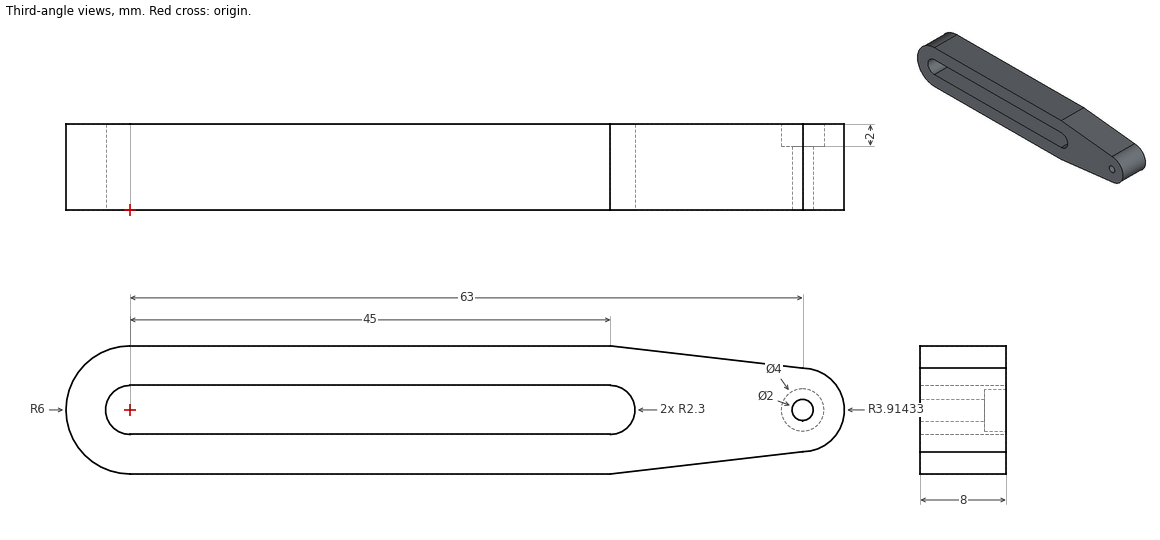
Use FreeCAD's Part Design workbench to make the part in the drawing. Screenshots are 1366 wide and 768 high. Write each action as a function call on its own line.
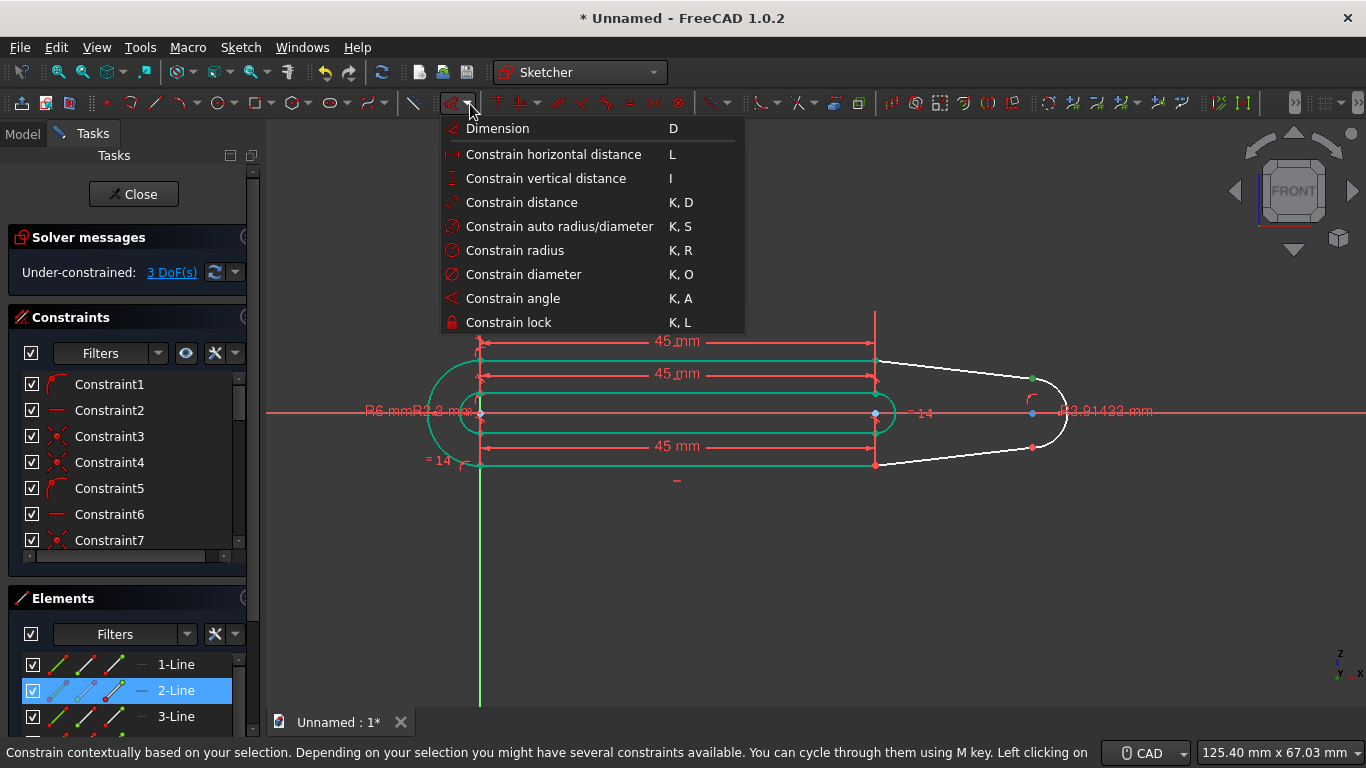
click(593, 154)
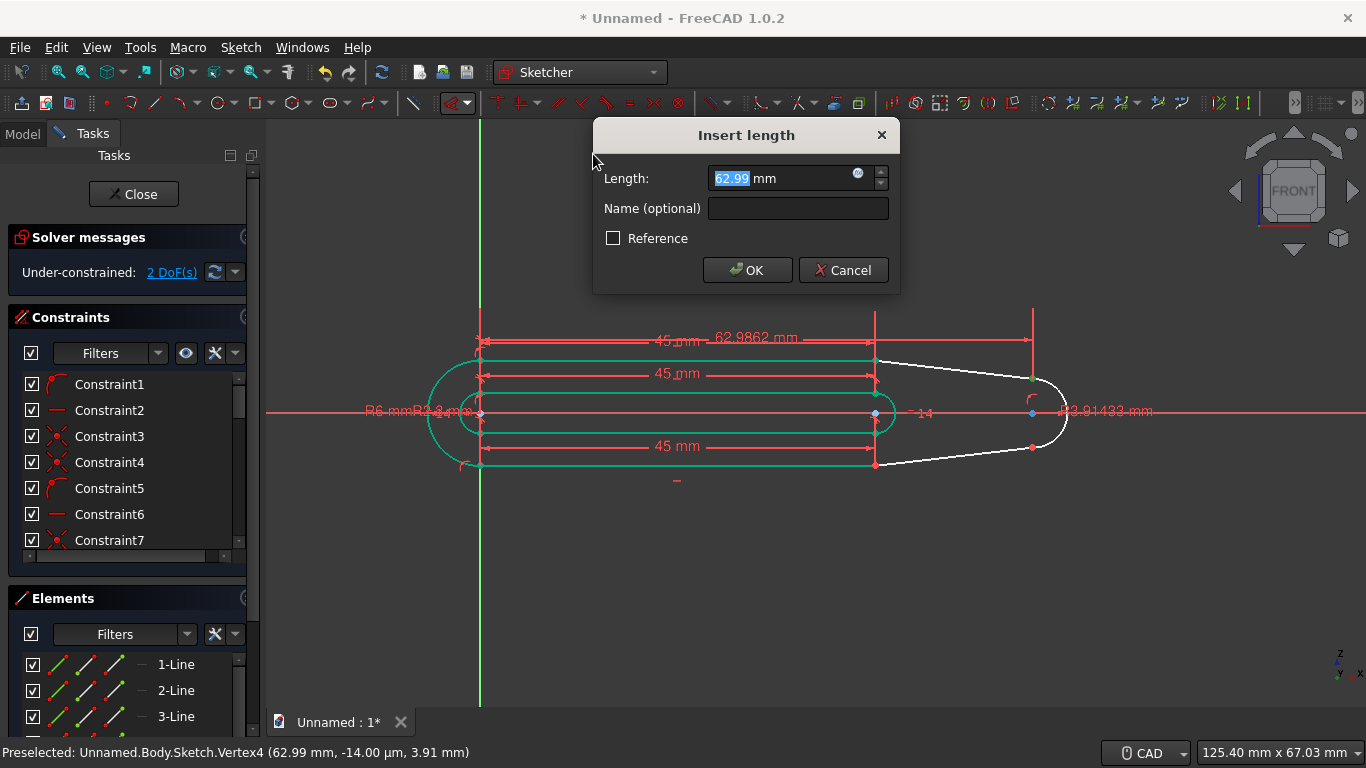
text(63)
key(Return)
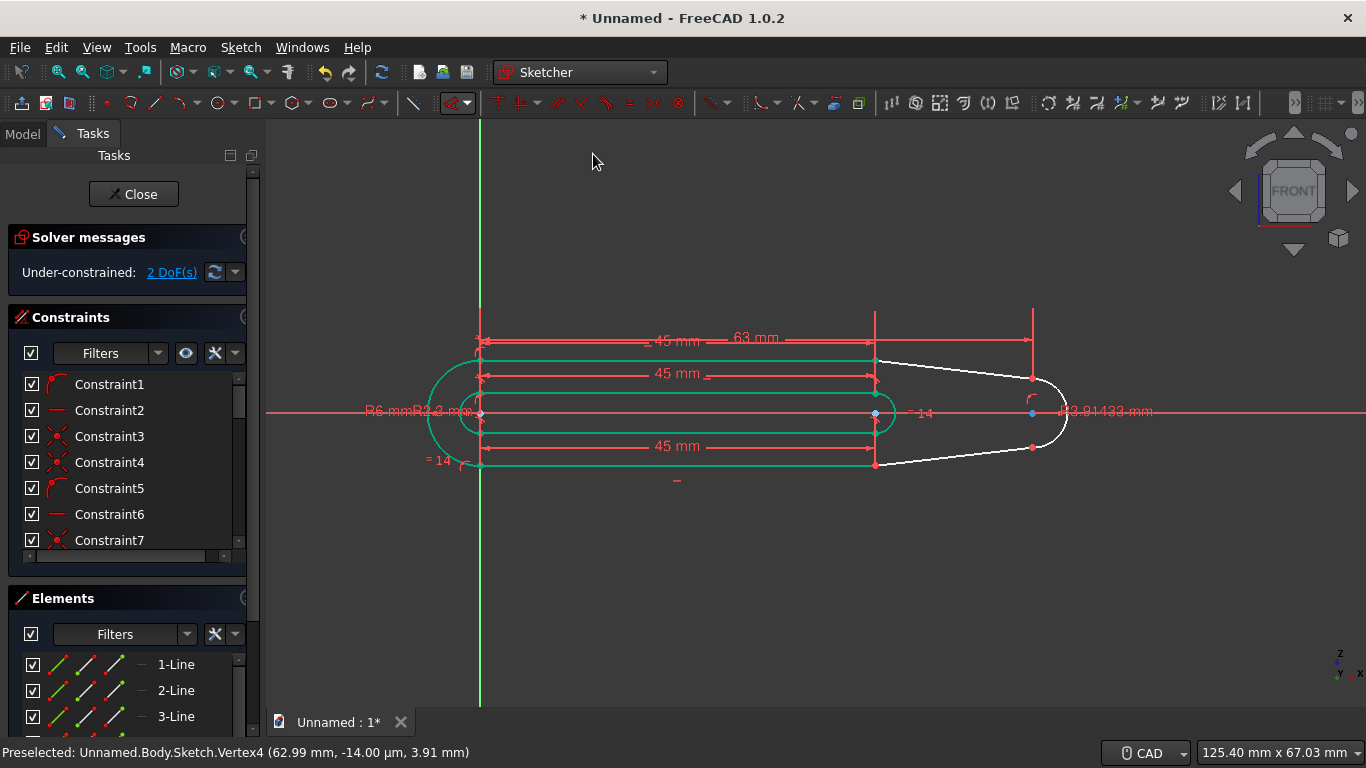
click(1033, 448)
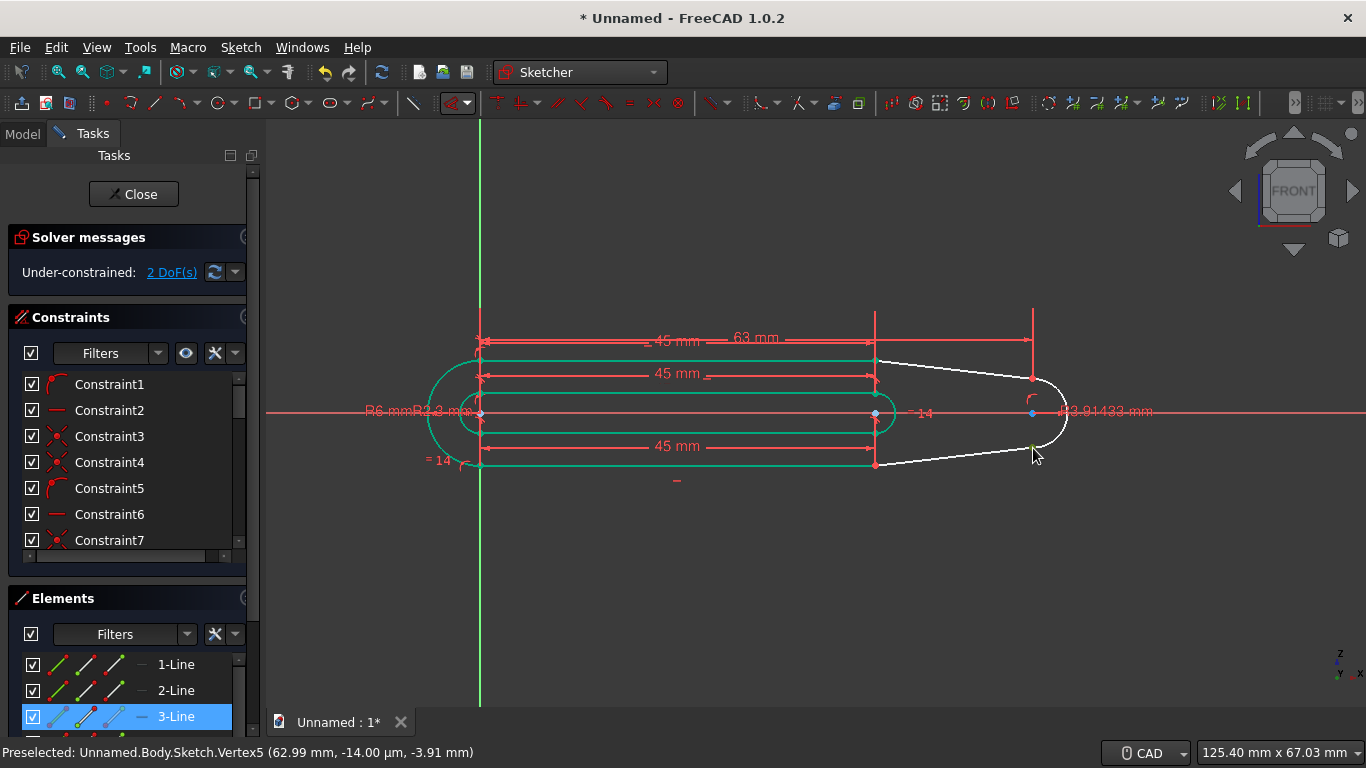
key(l)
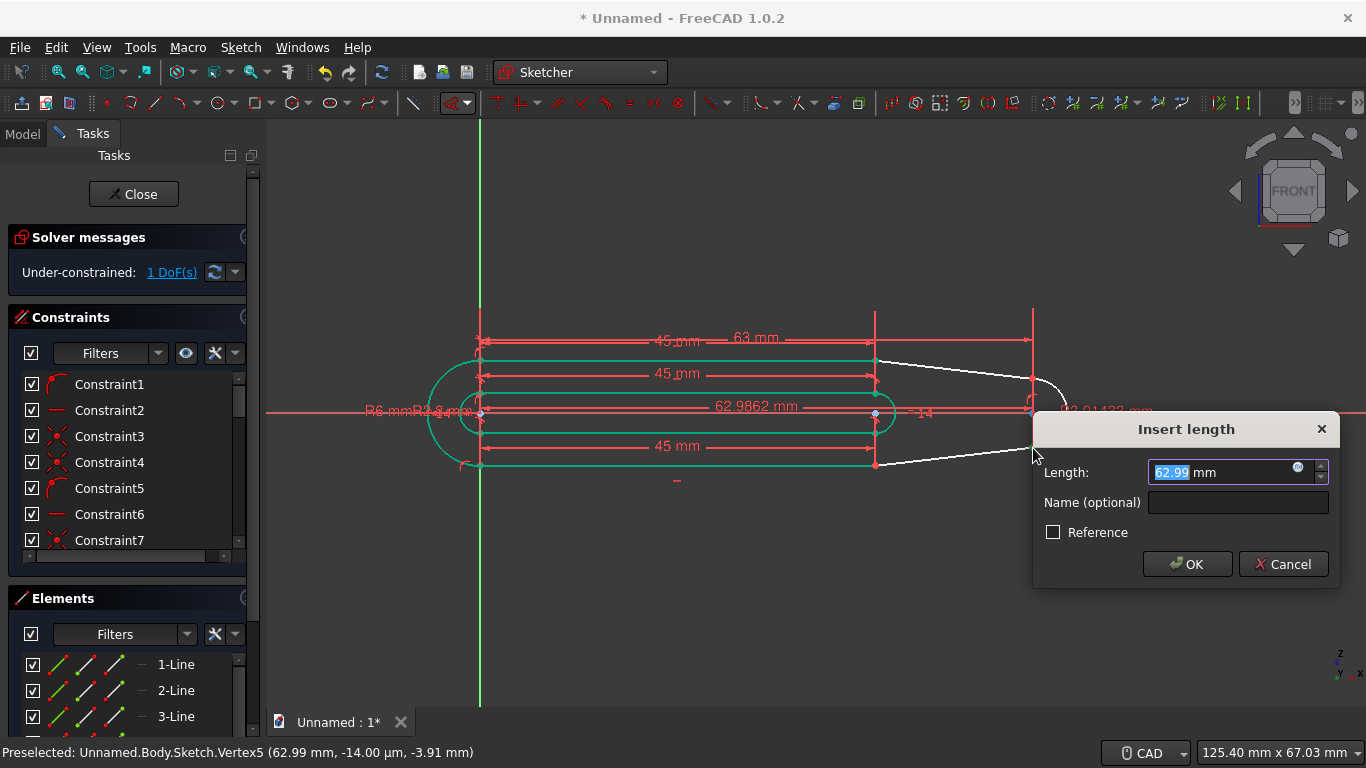
text(63)
key(Return)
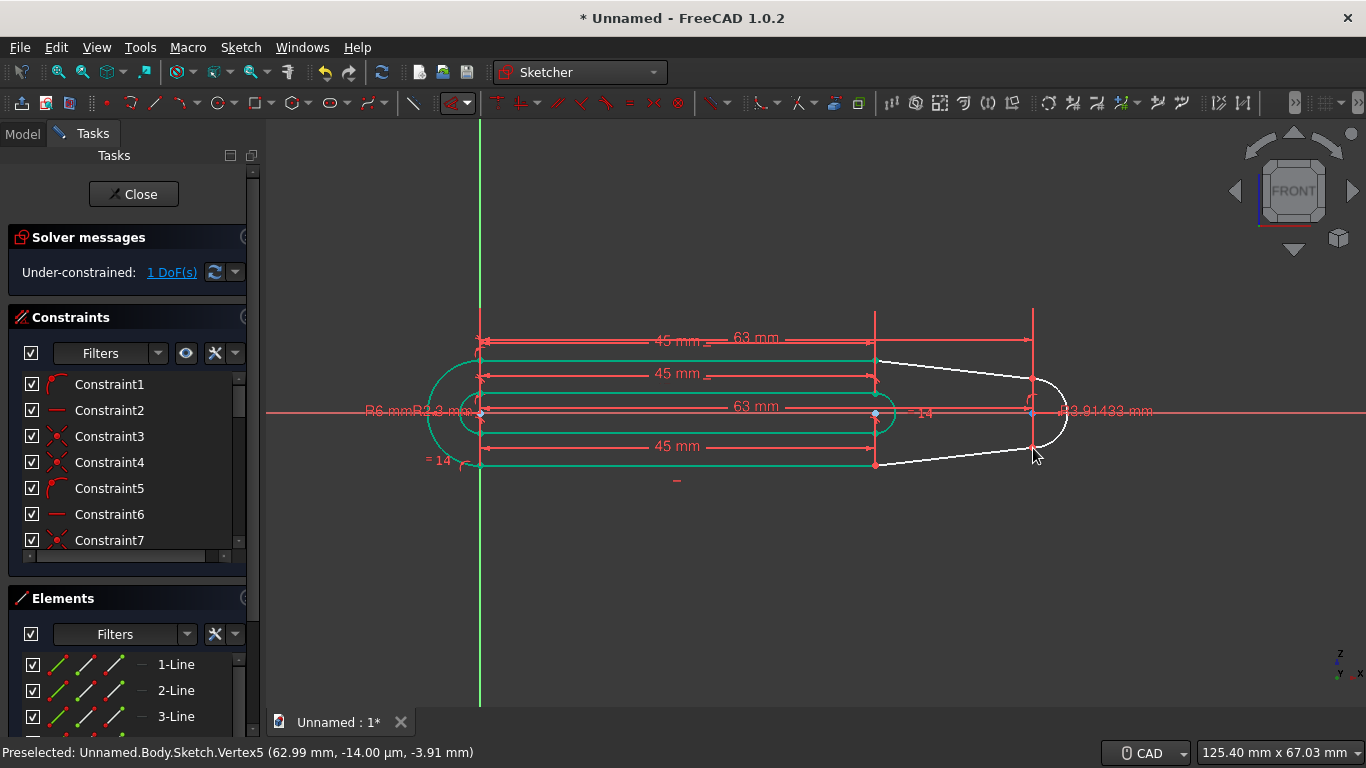
click(1033, 413)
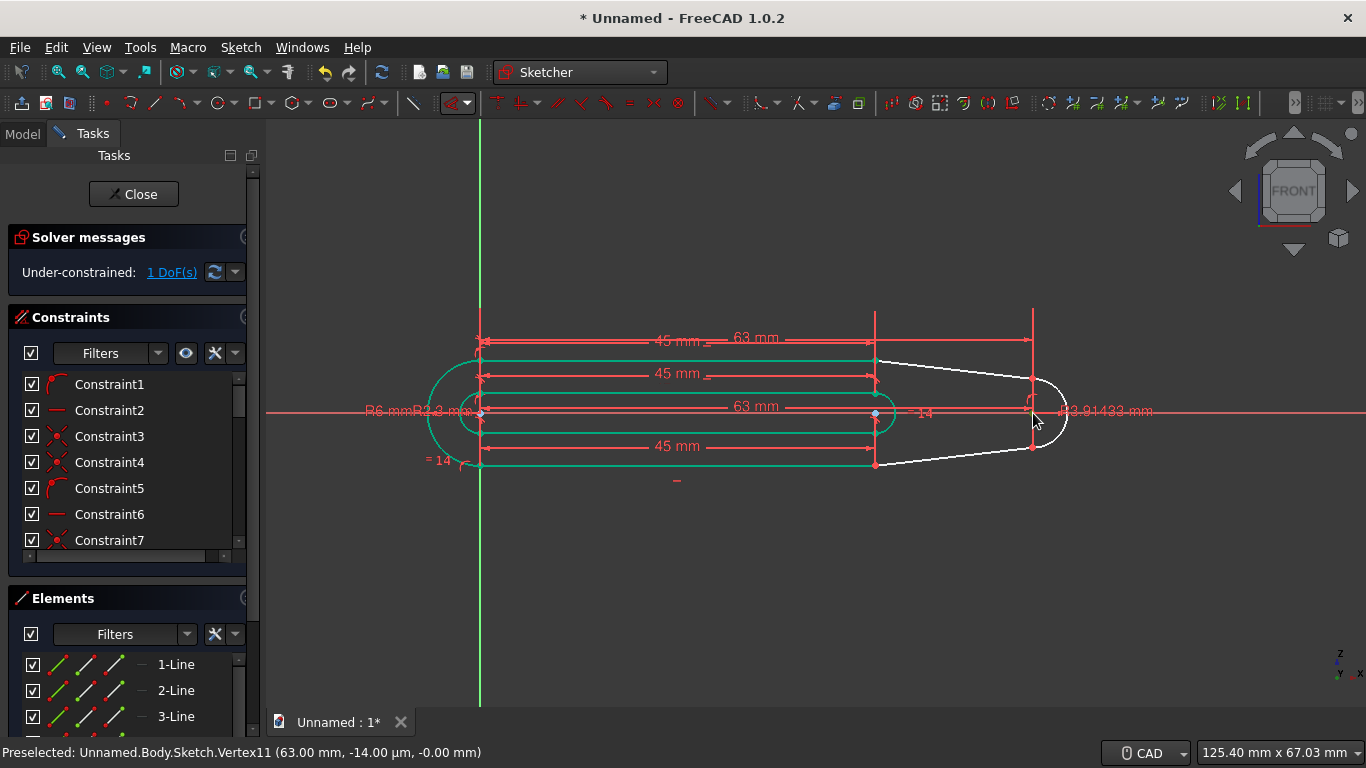
click(470, 104)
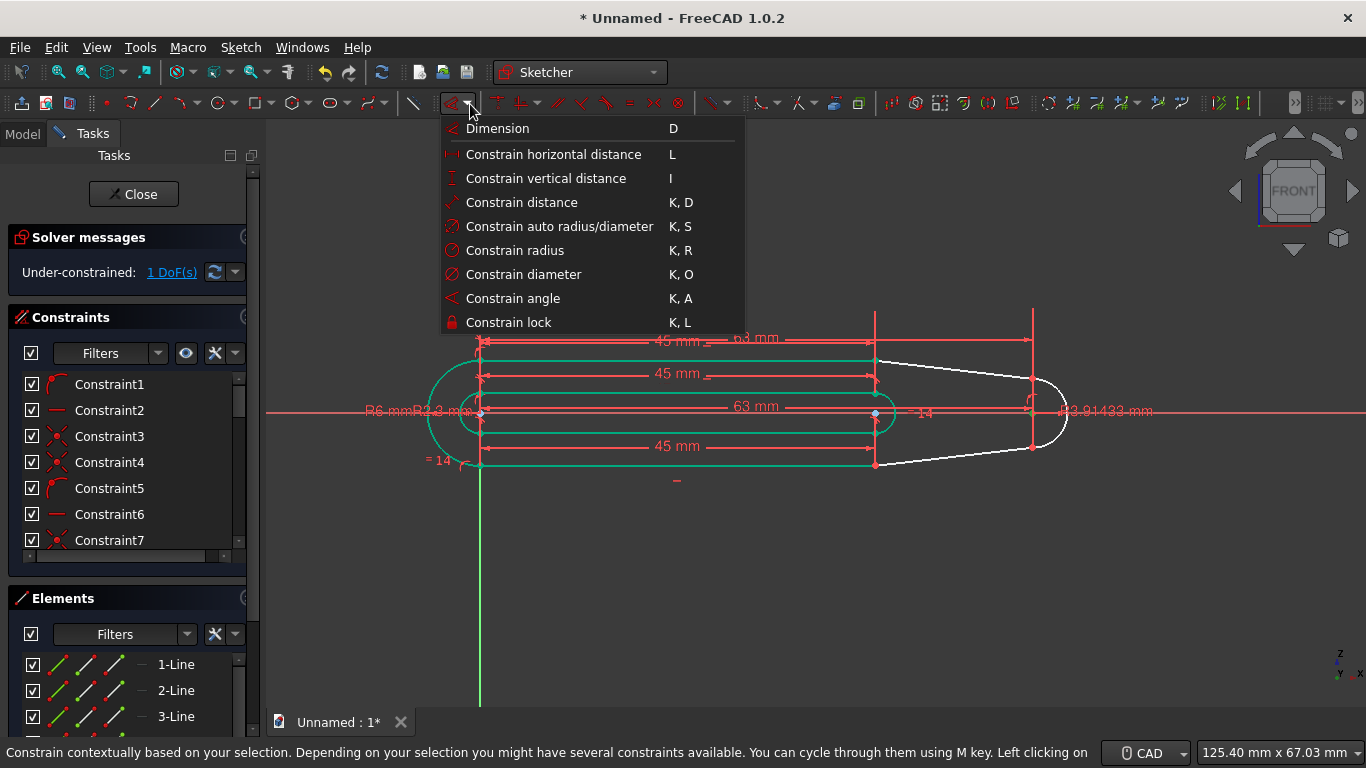
click(593, 154)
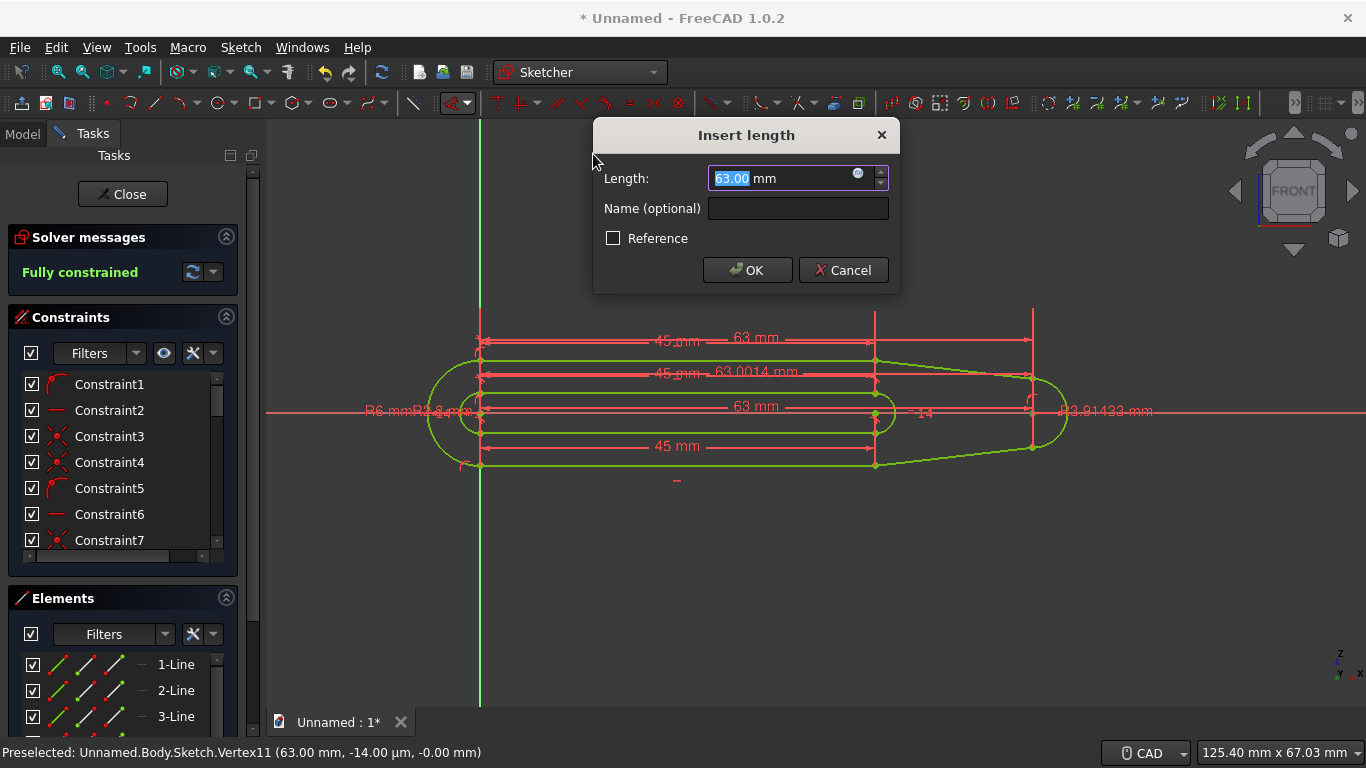
text(63)
key(Return)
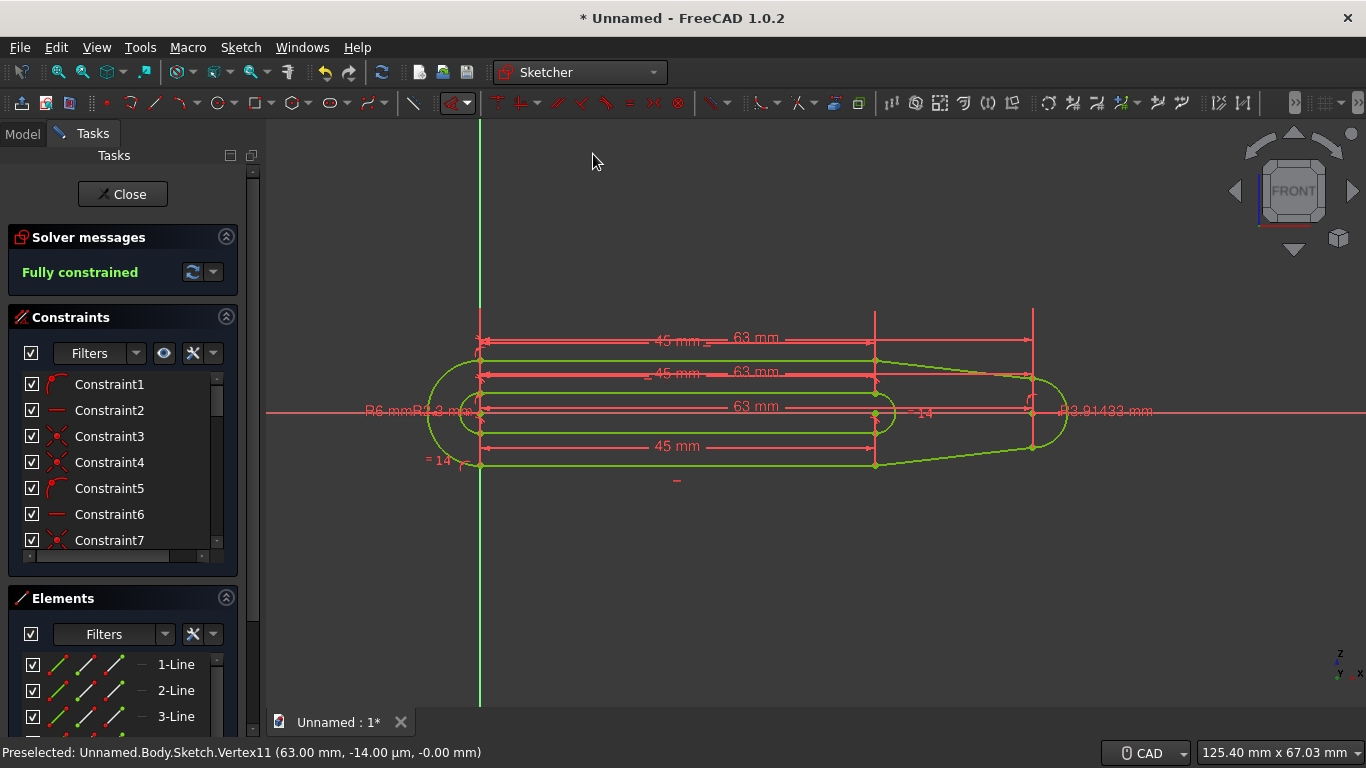
click(123, 194)